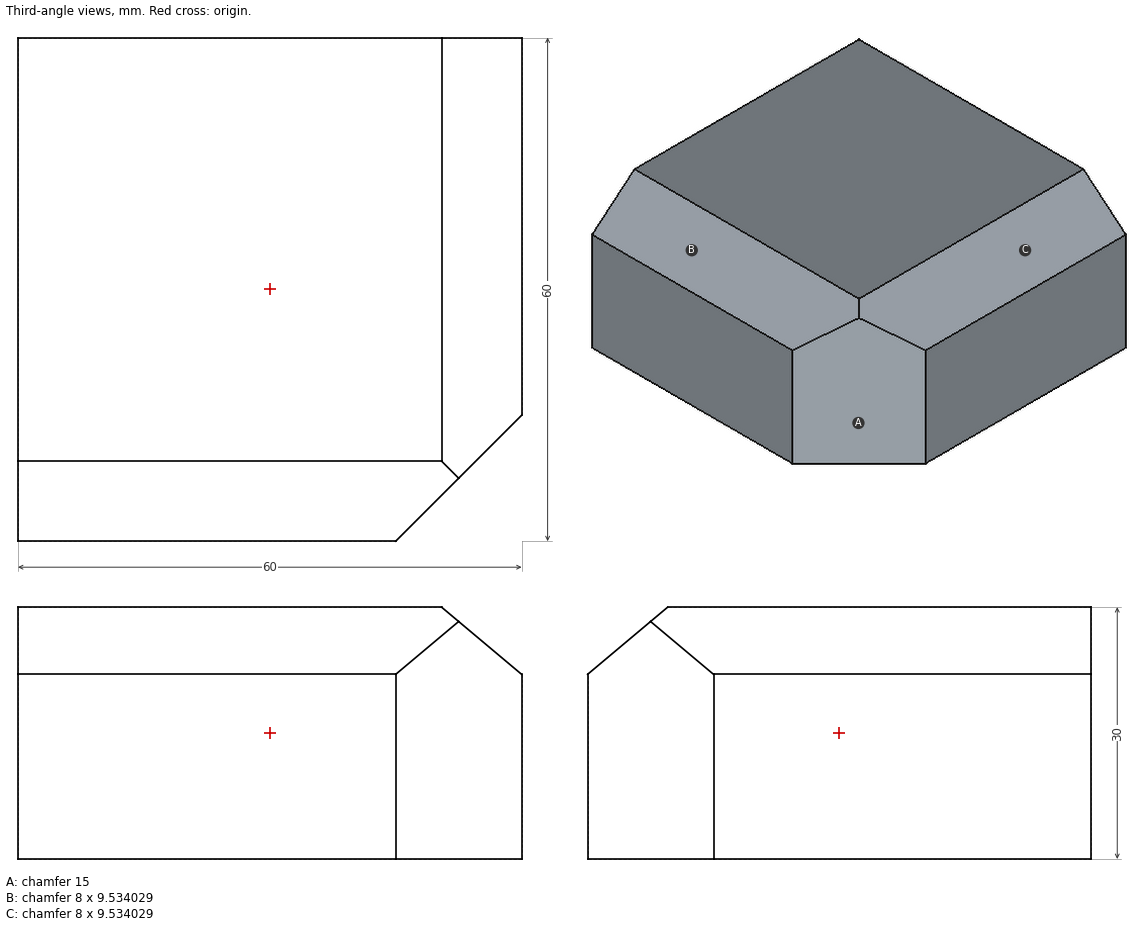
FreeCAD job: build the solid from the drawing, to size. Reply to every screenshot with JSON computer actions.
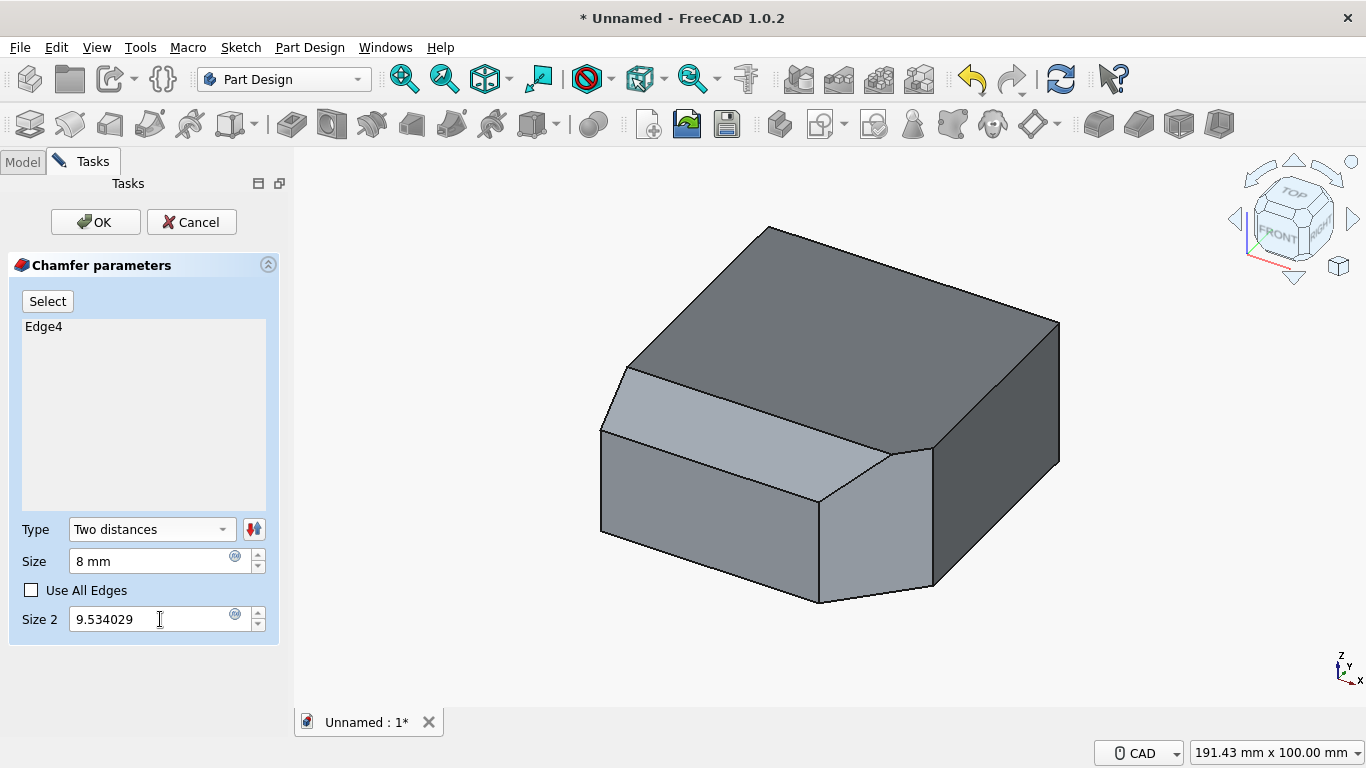
{"action": "left_click", "coordinate": [96, 222]}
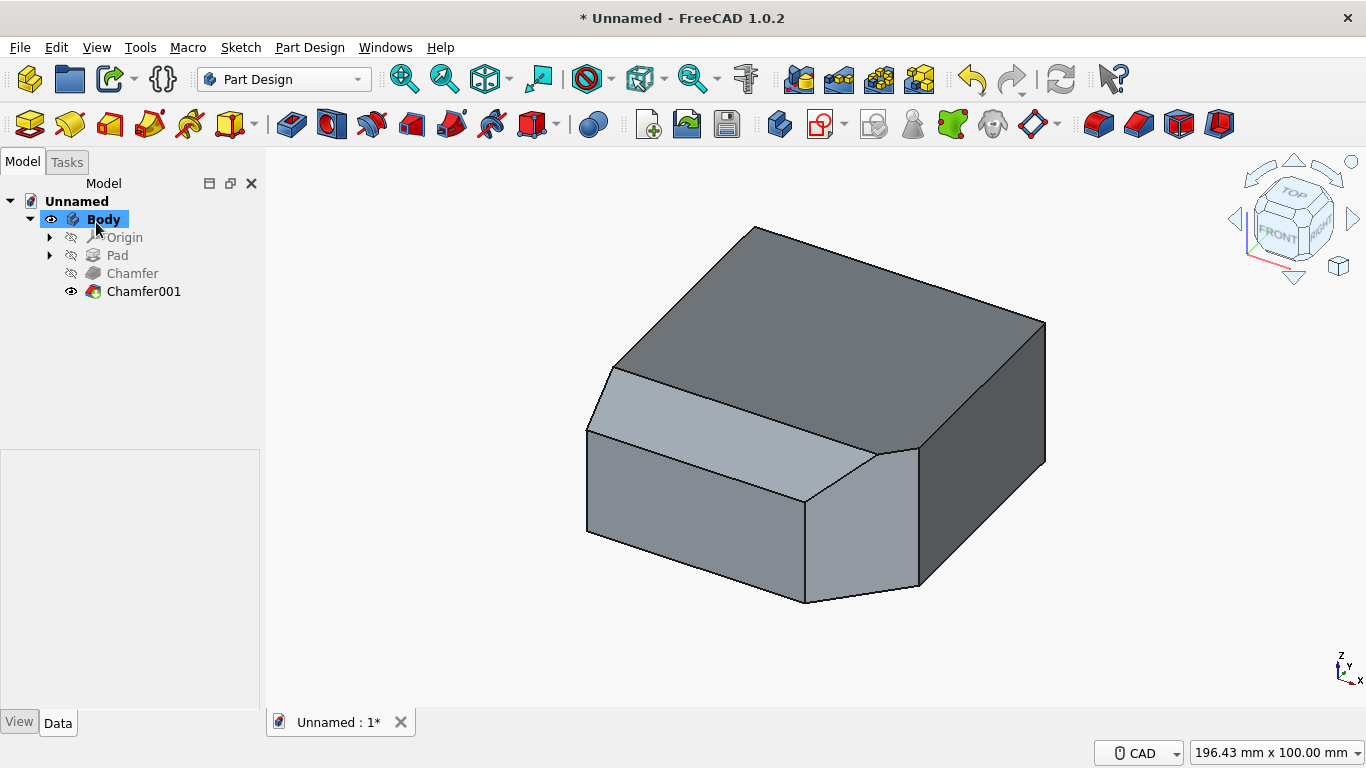
{"action": "left_click", "coordinate": [982, 385]}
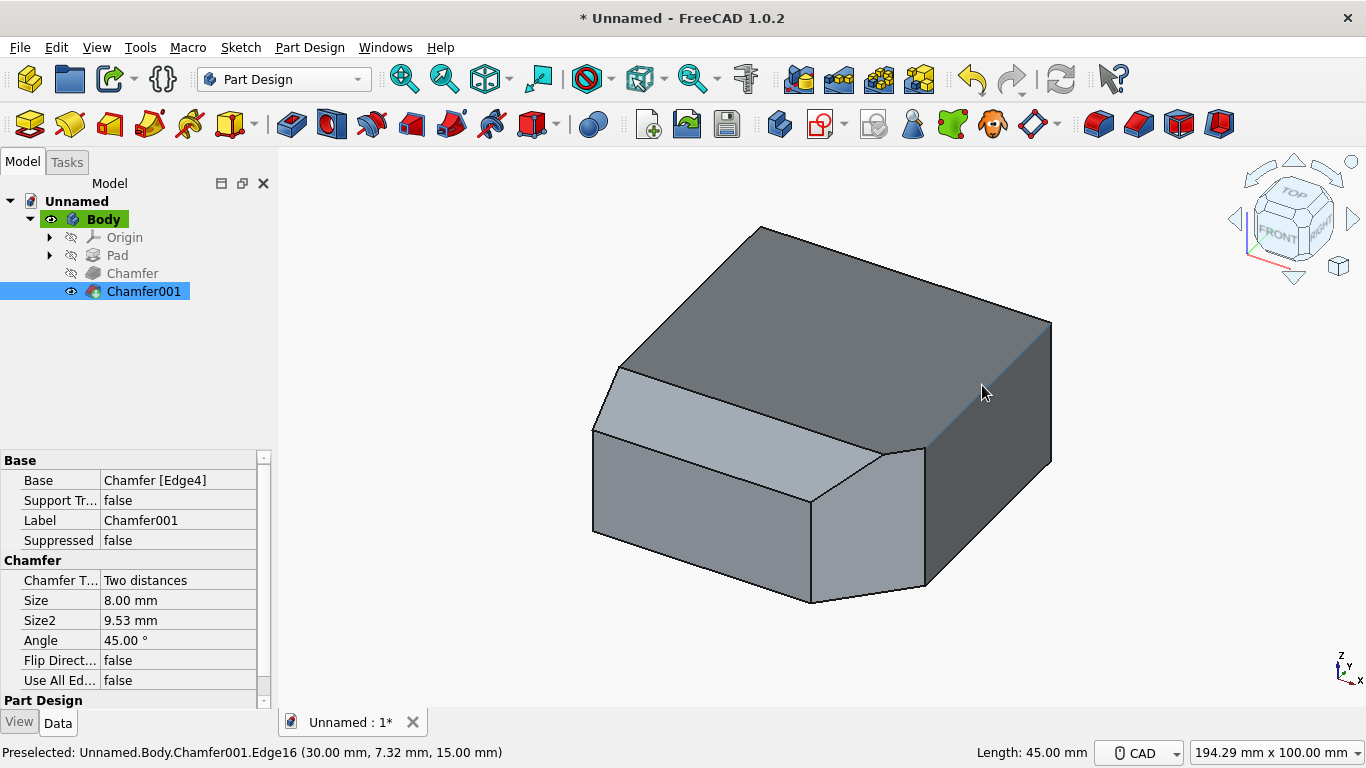
{"action": "left_click", "coordinate": [1140, 124]}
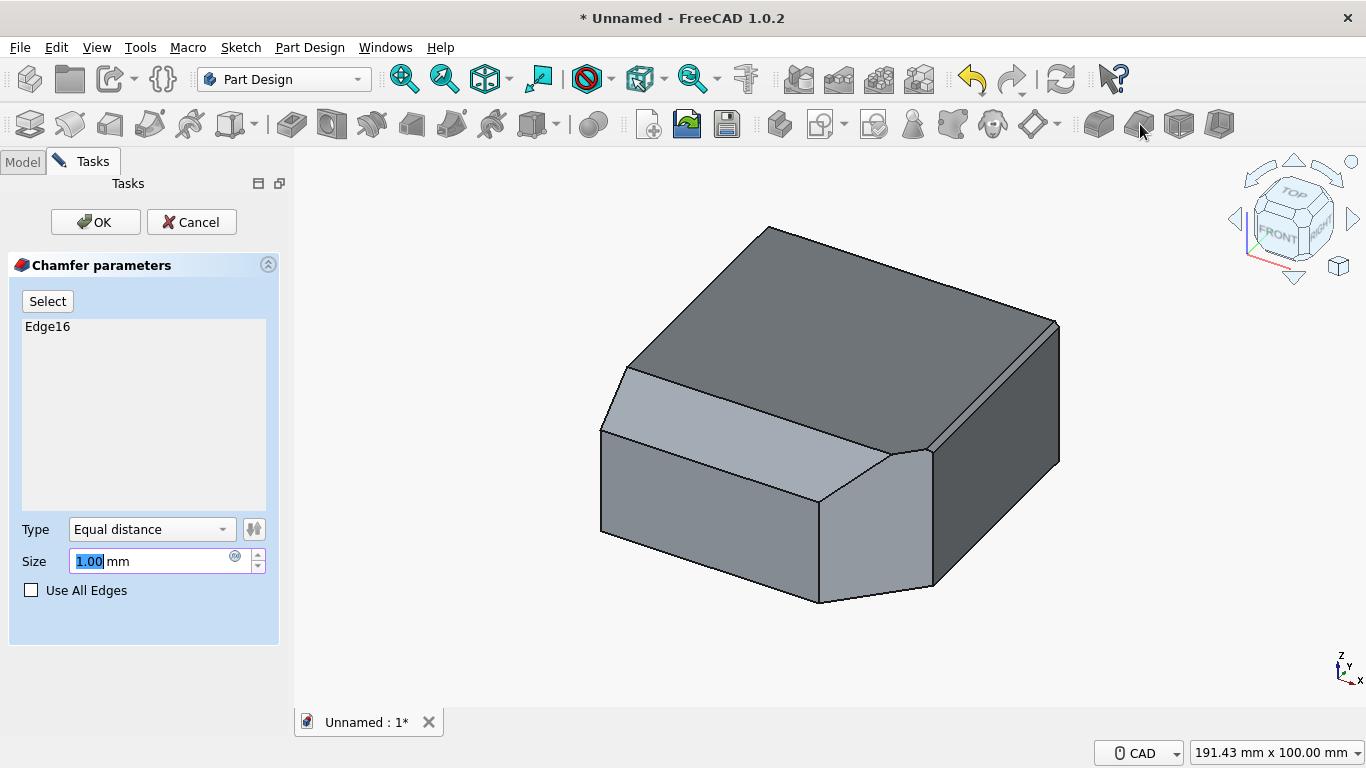
{"action": "type", "text": "8"}
{"action": "key", "text": "Tab"}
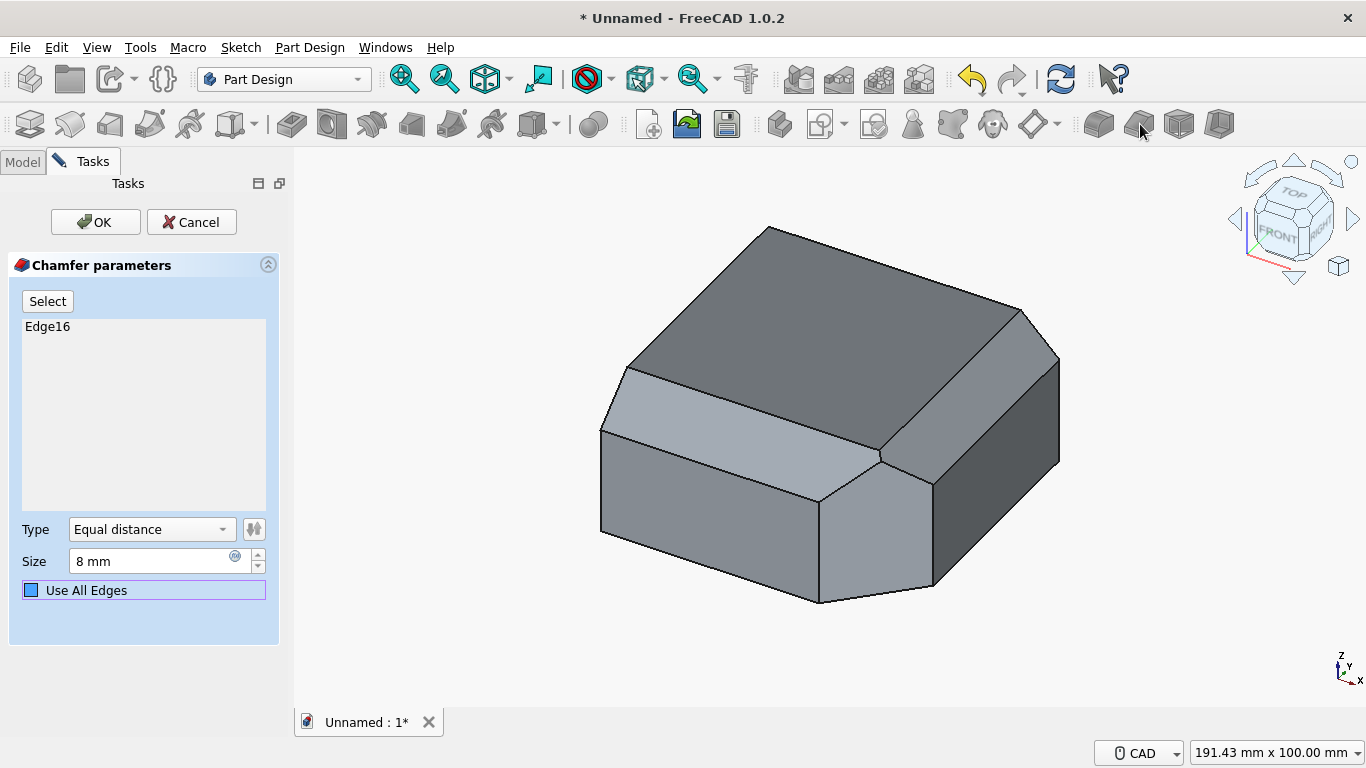
{"action": "left_click", "coordinate": [153, 530]}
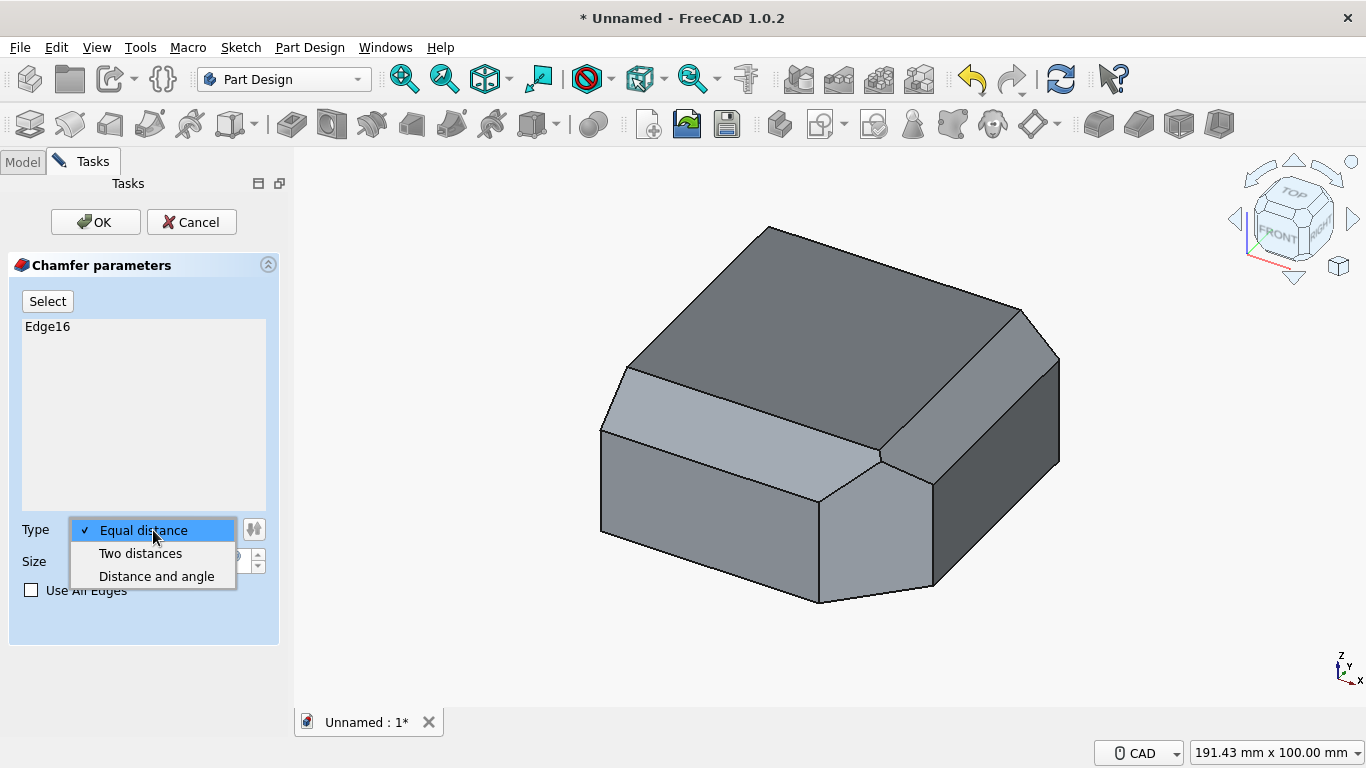
{"action": "left_click", "coordinate": [152, 554]}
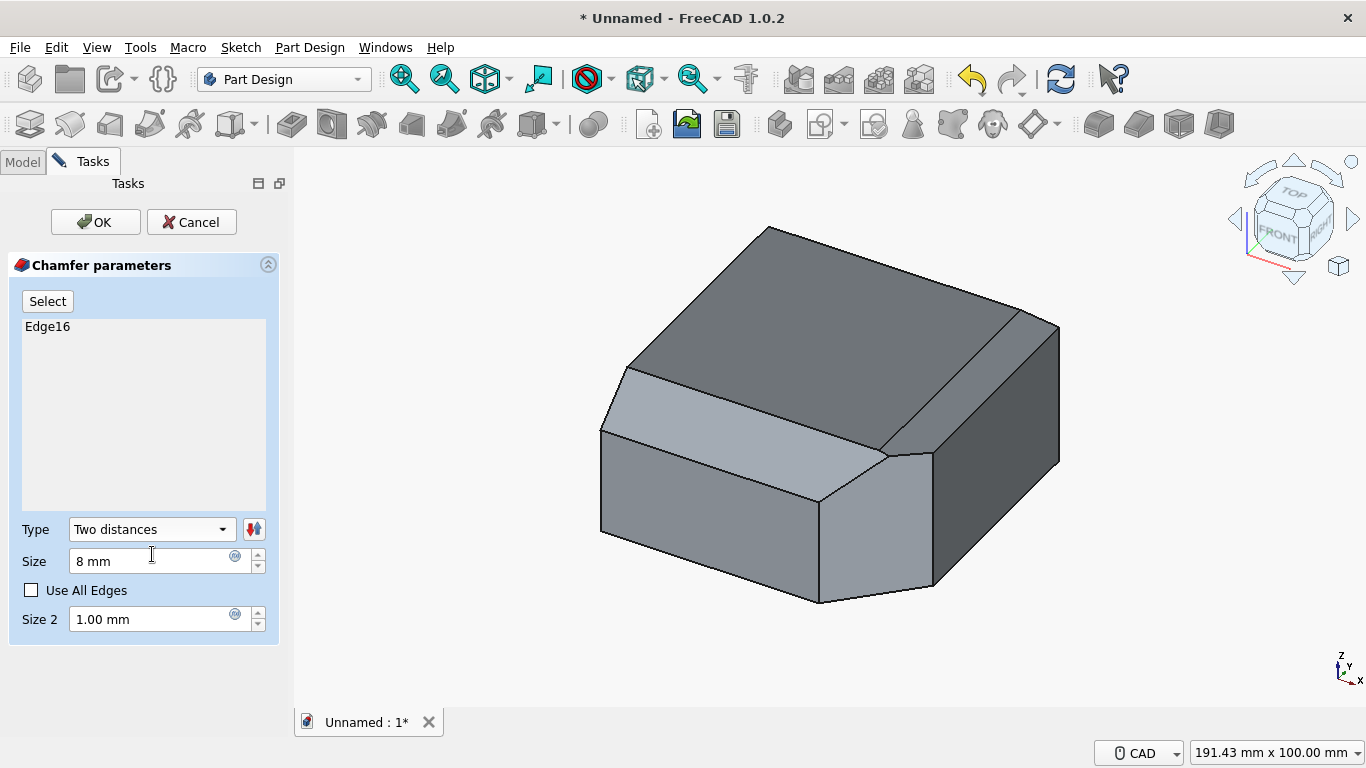
{"action": "triple_click", "coordinate": [160, 619]}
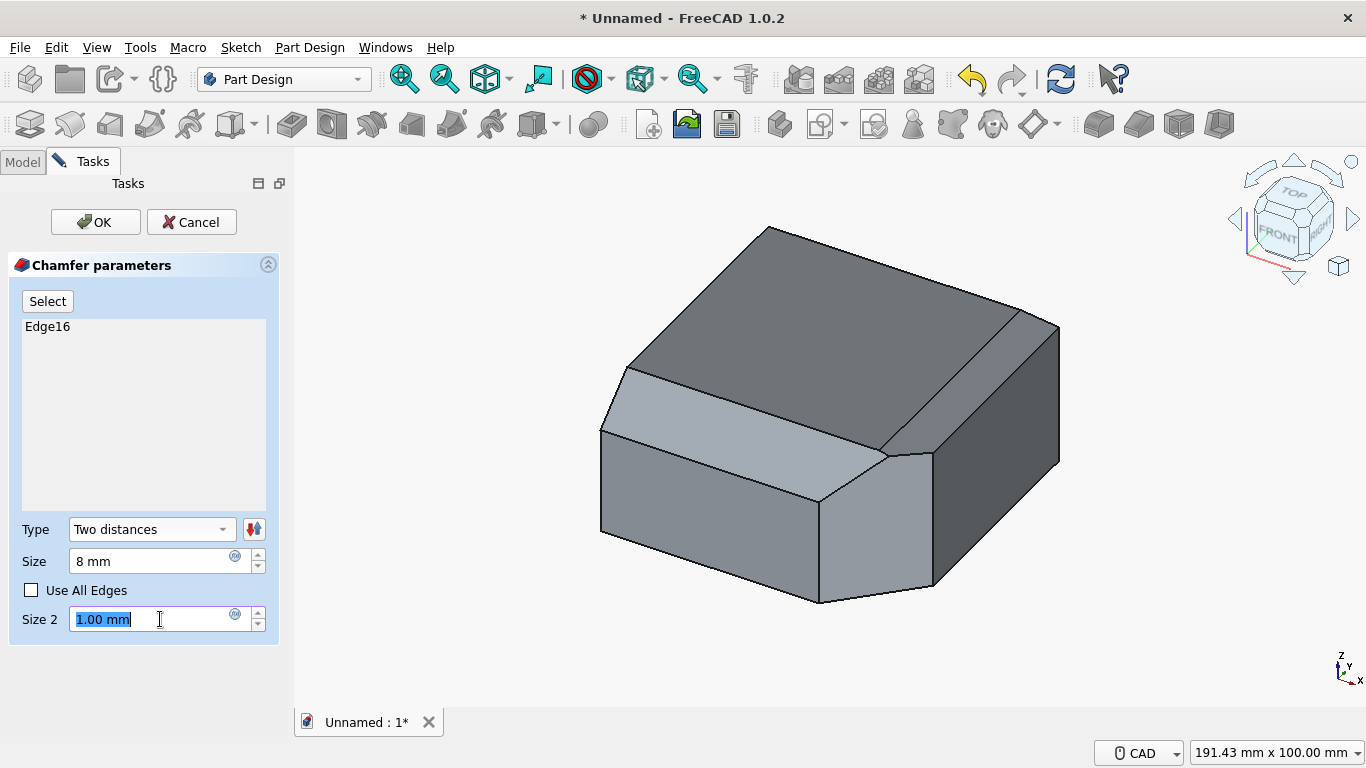
{"action": "type", "text": "9.534029"}
{"action": "key", "text": "Tab"}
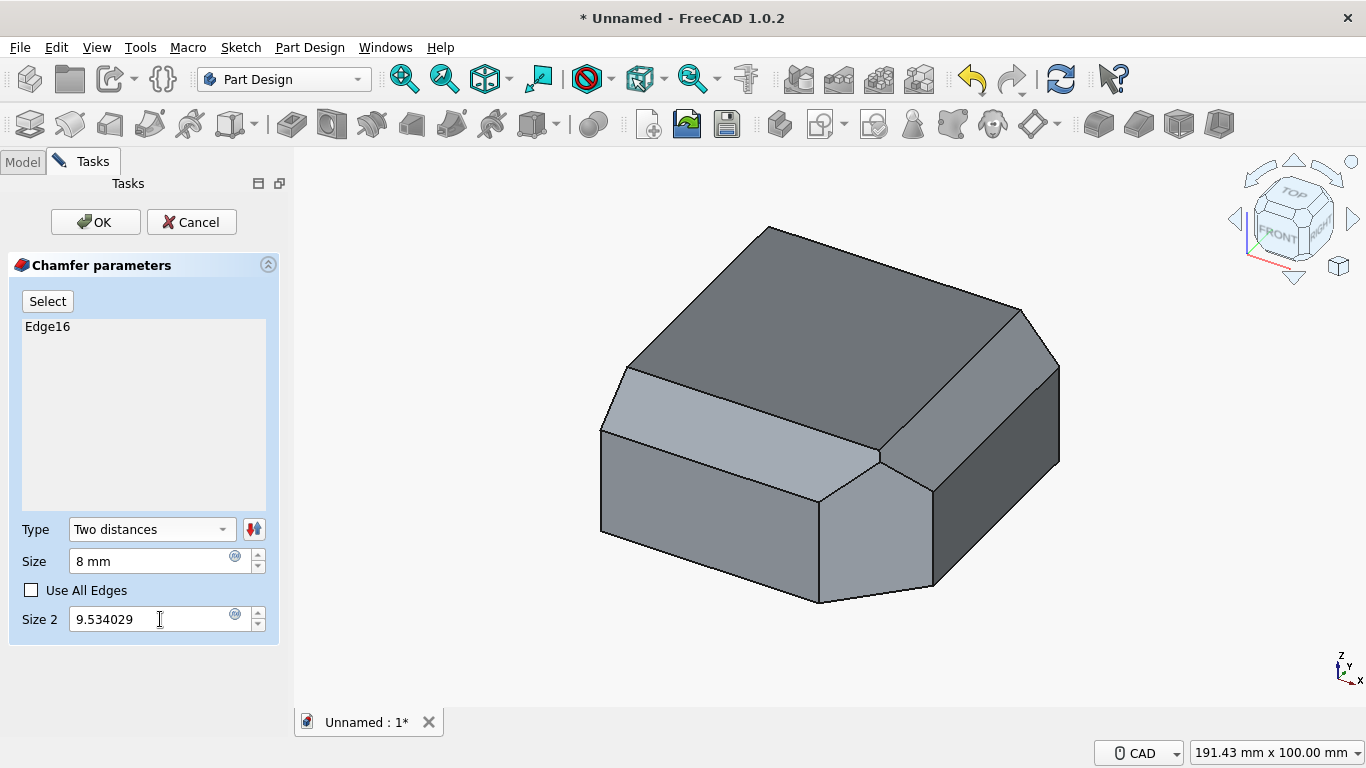
{"action": "left_click", "coordinate": [254, 530]}